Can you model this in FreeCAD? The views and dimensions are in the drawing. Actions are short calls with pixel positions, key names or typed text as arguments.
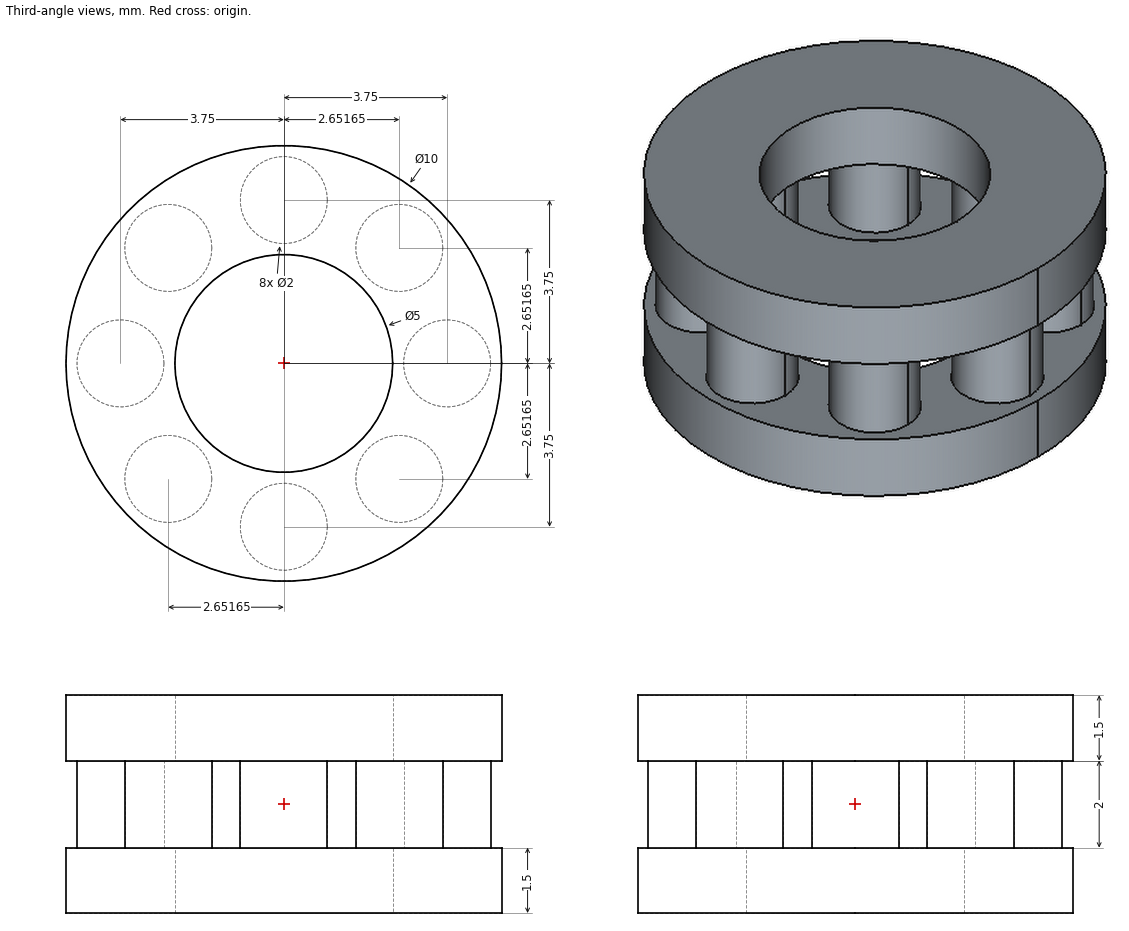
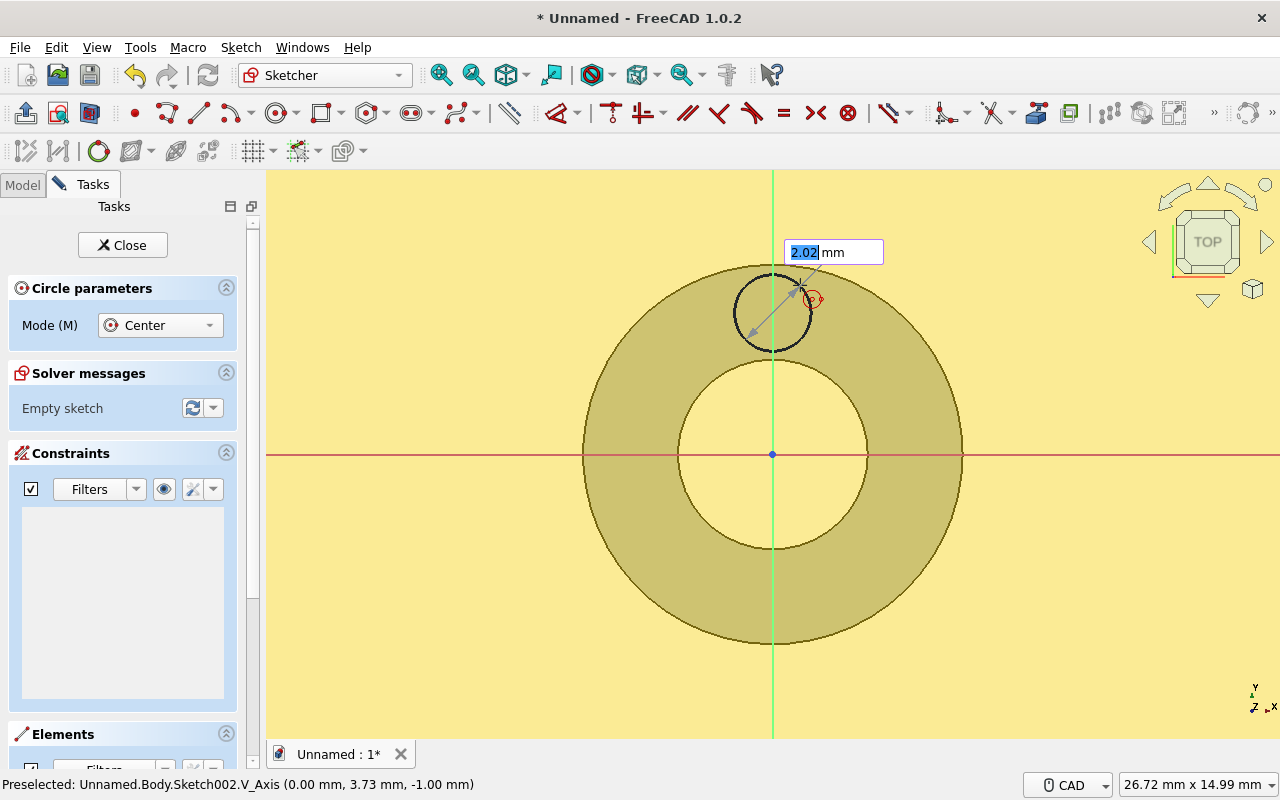
text(2)
key(Return)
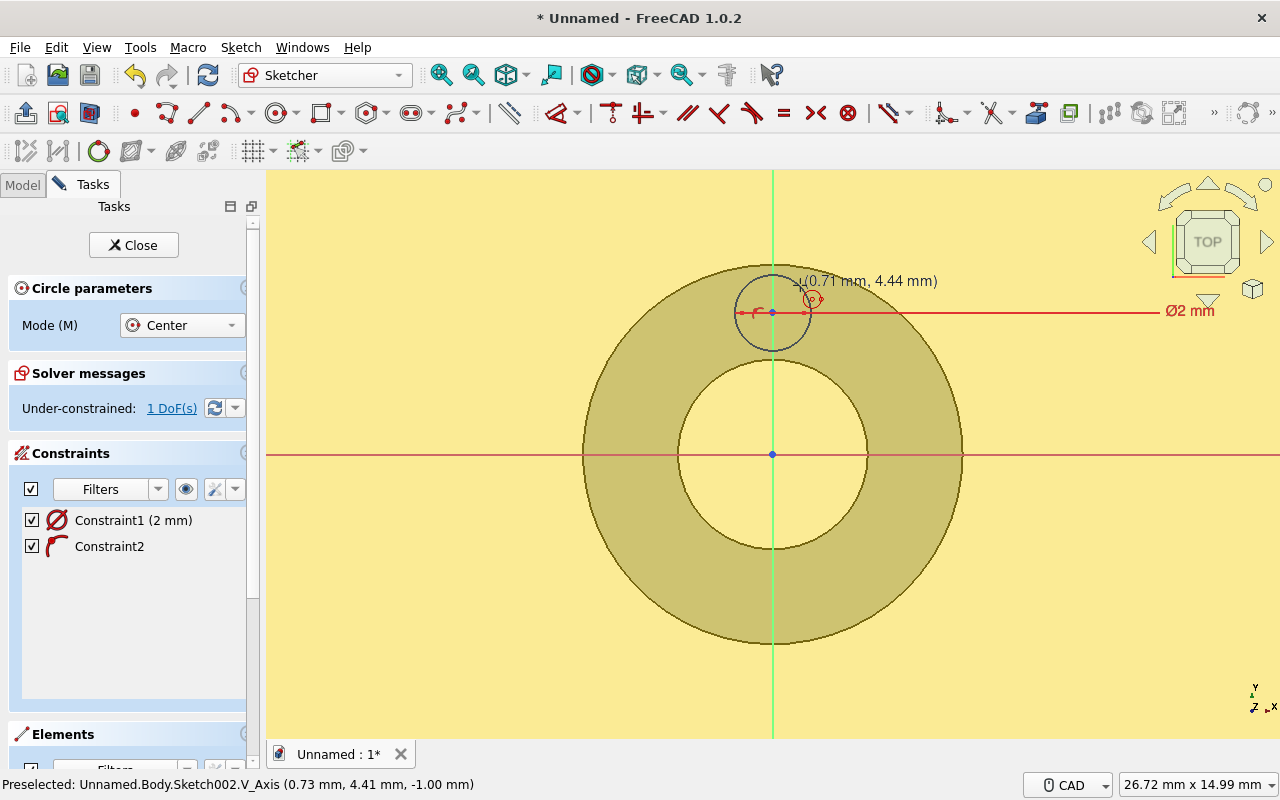
click(873, 354)
move(900, 327)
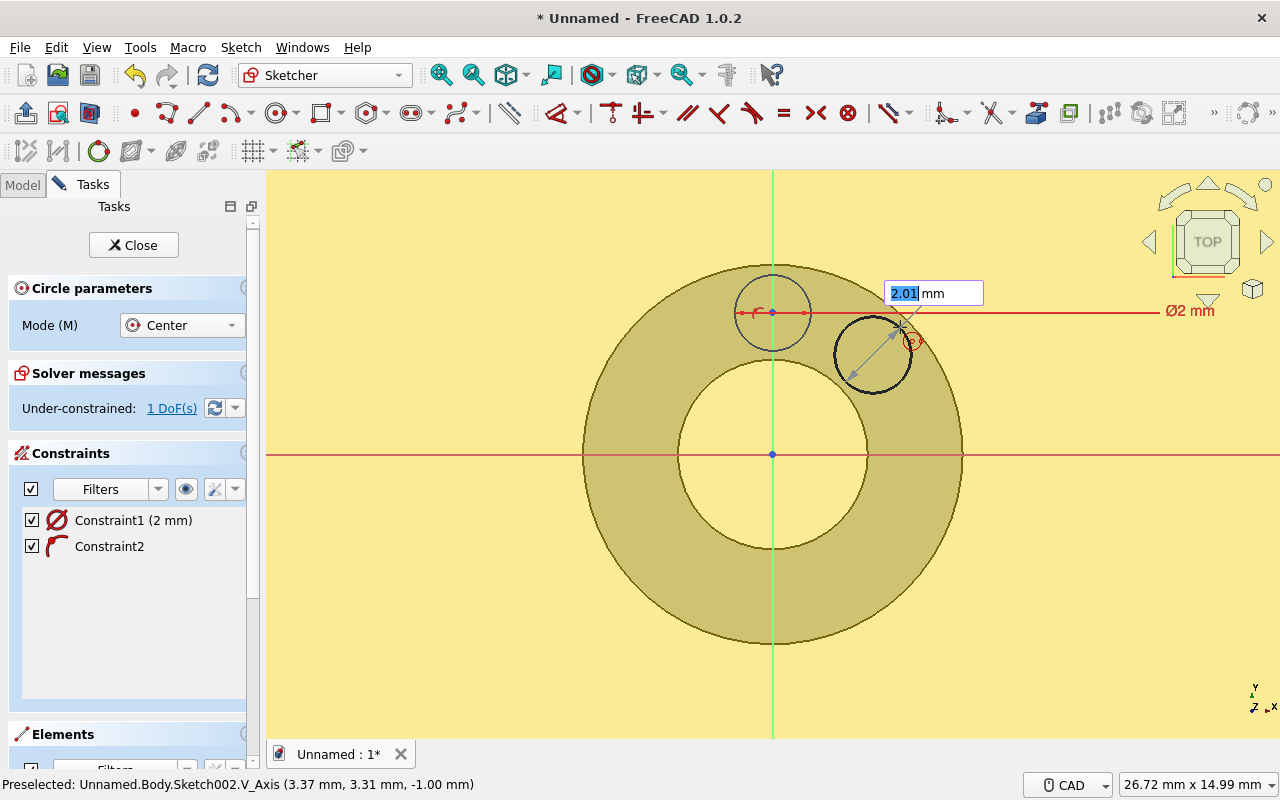
text(2)
key(Return)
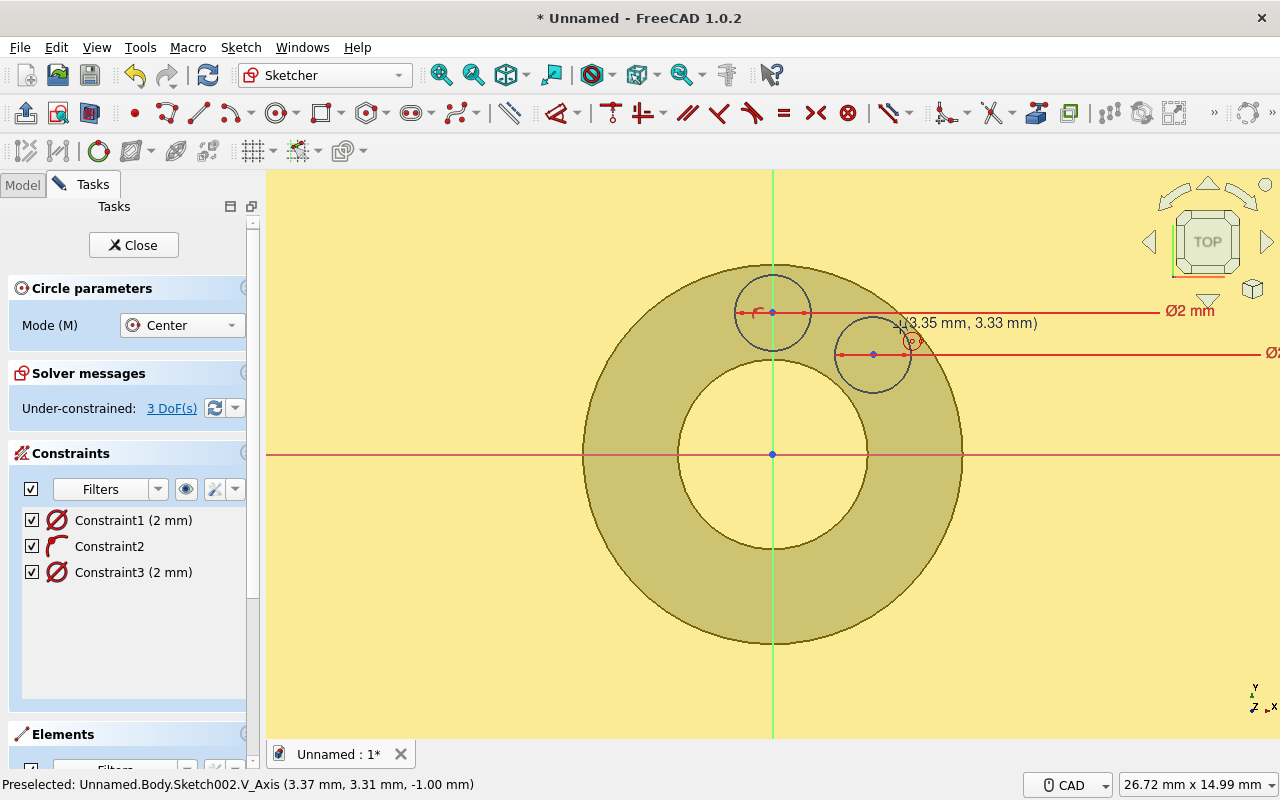
click(915, 454)
move(942, 428)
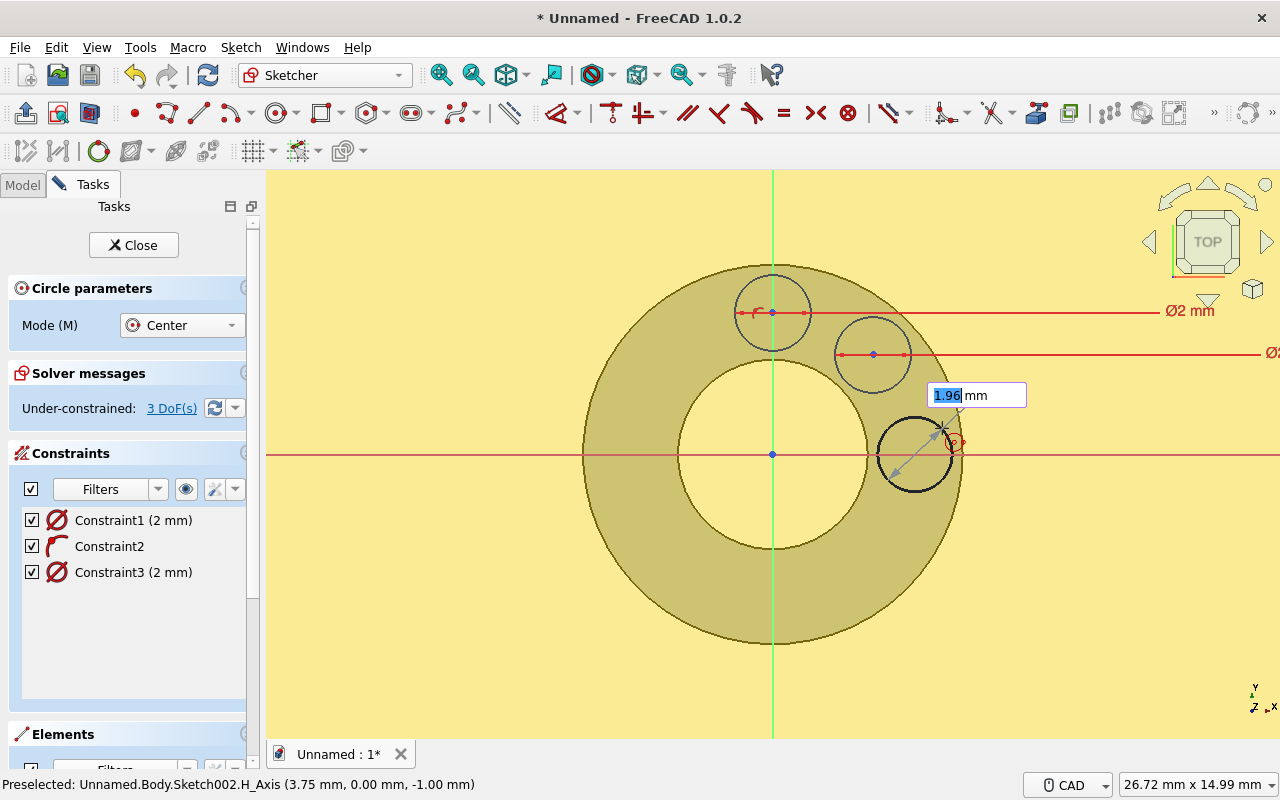
text(2)
key(Return)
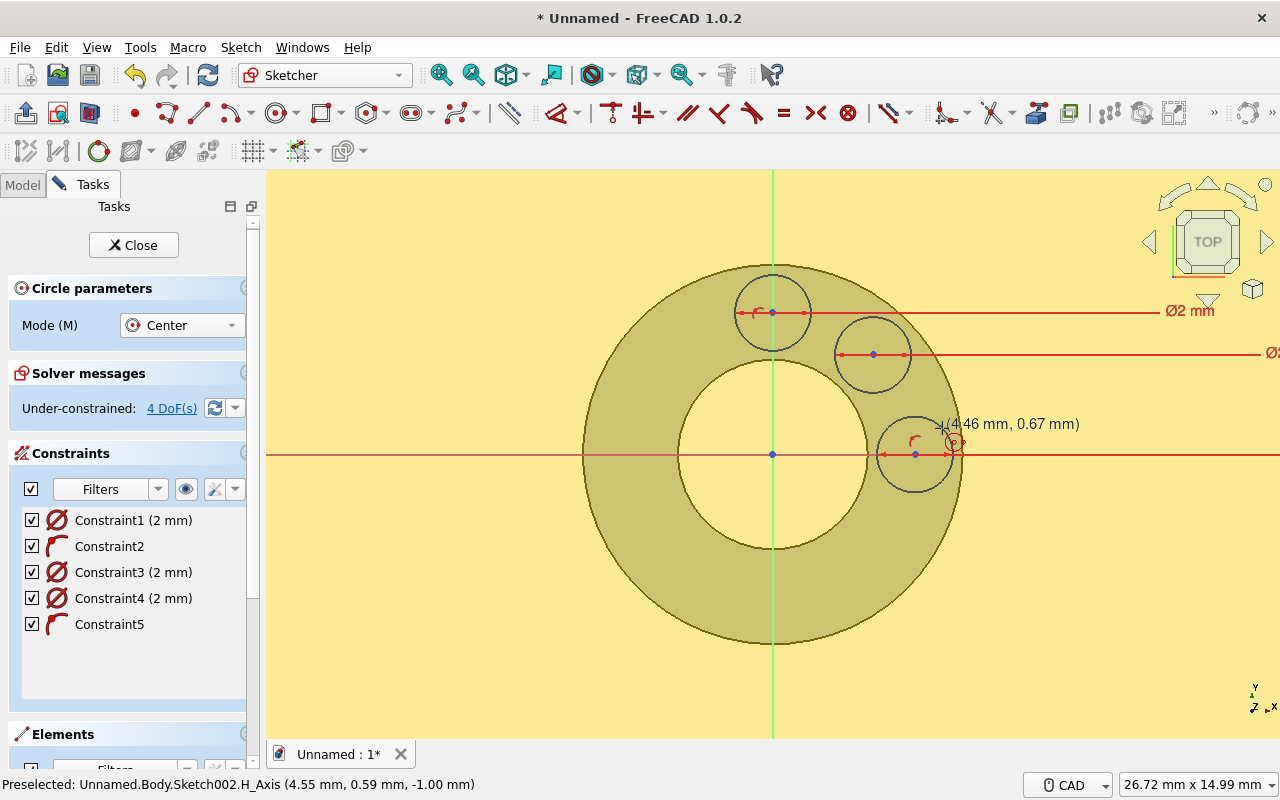
click(873, 555)
move(900, 528)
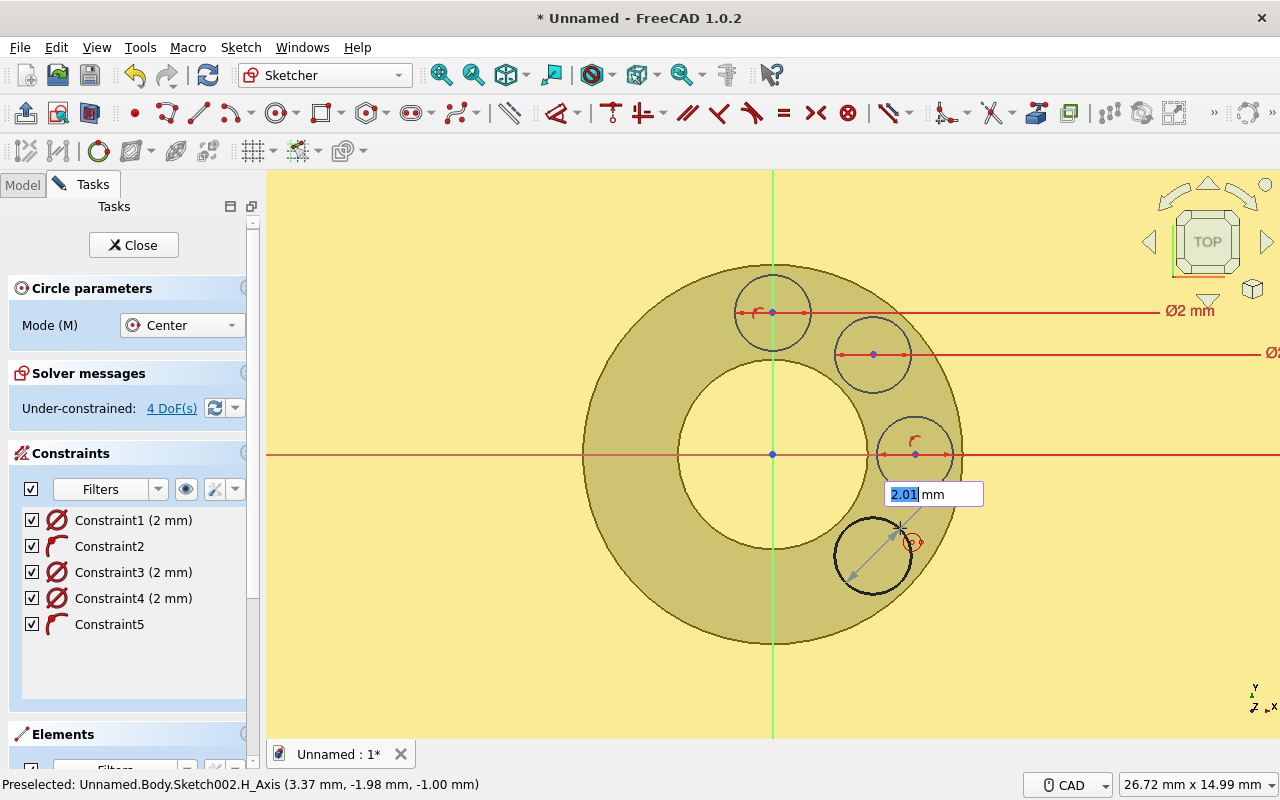
text(2)
key(Return)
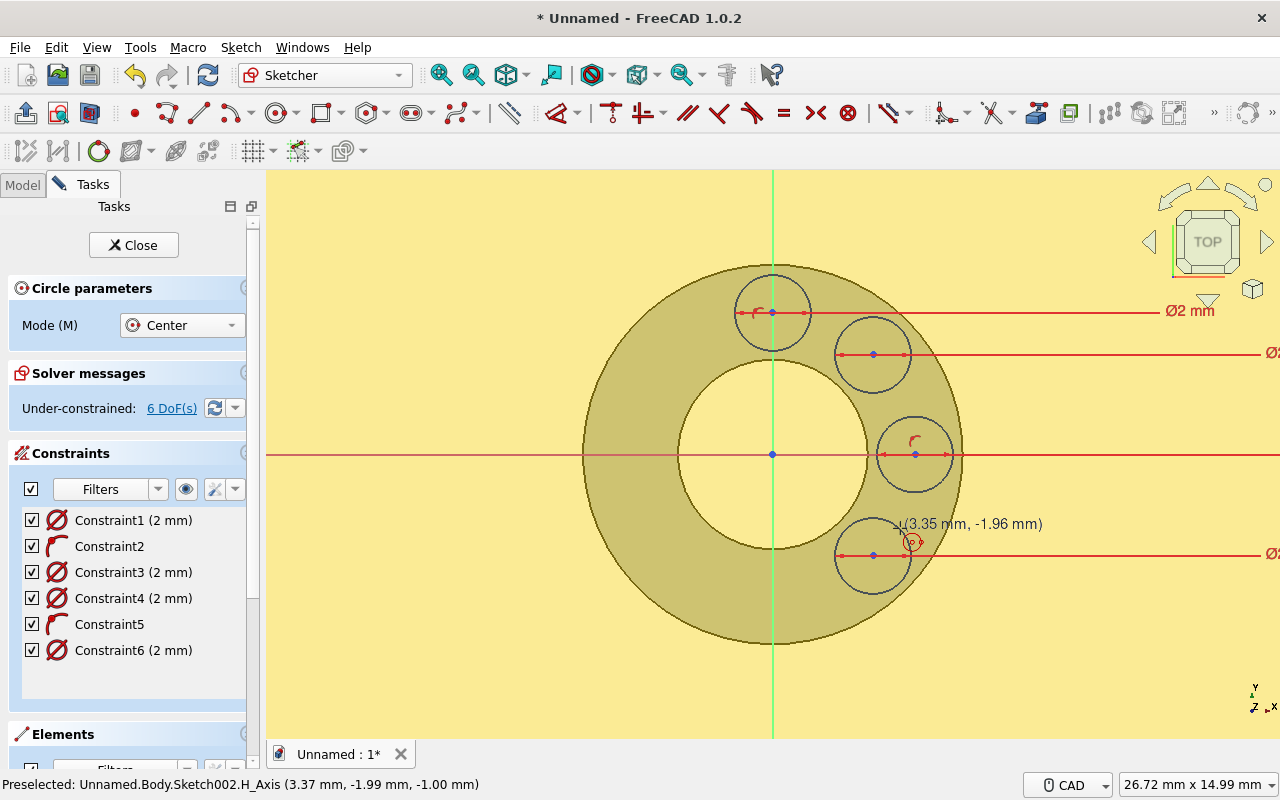
click(773, 597)
move(800, 570)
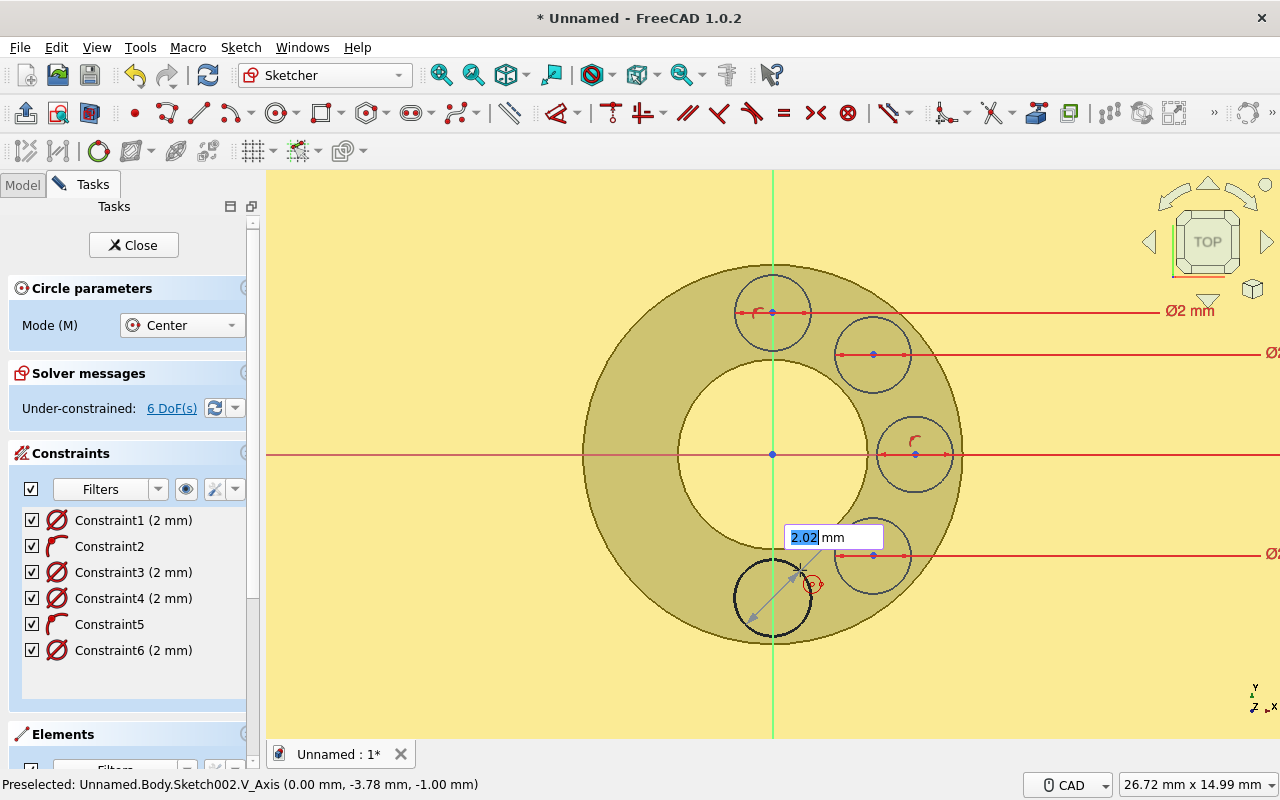
text(2)
key(Return)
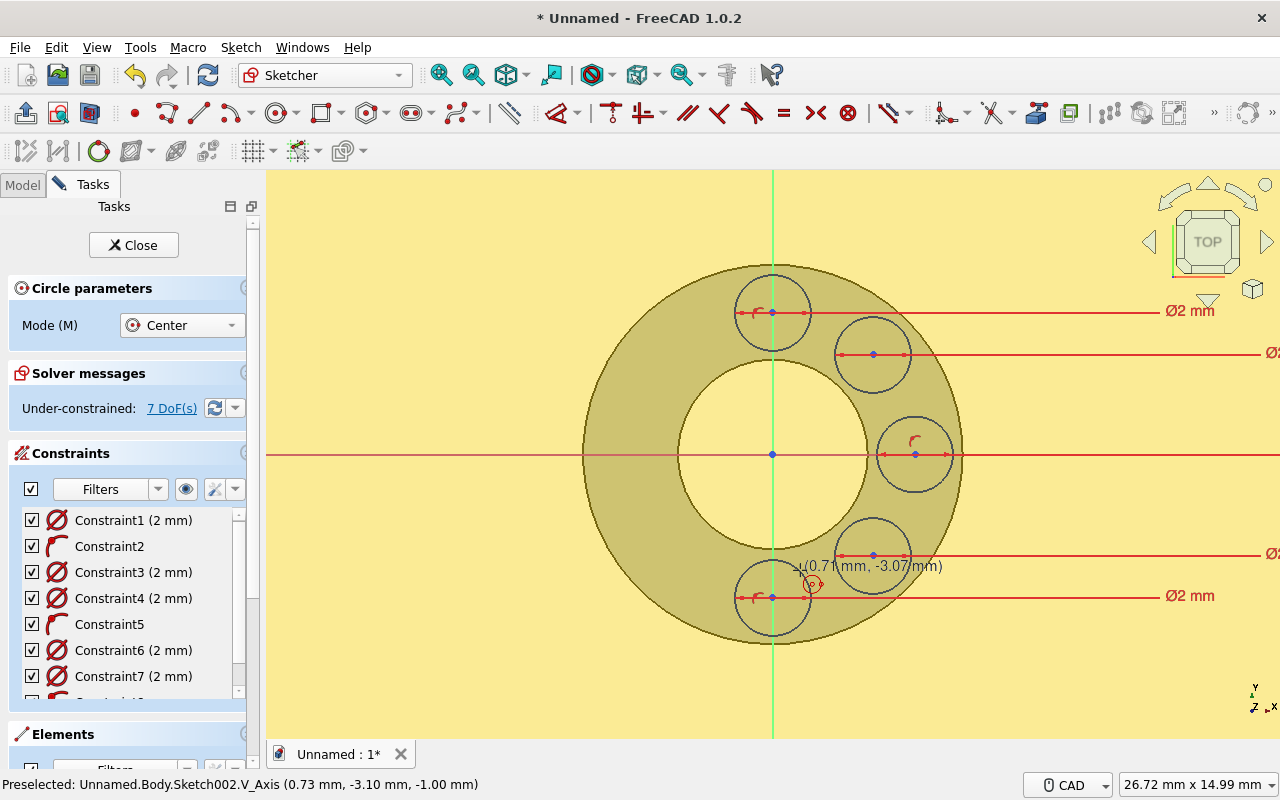
click(672, 555)
move(699, 528)